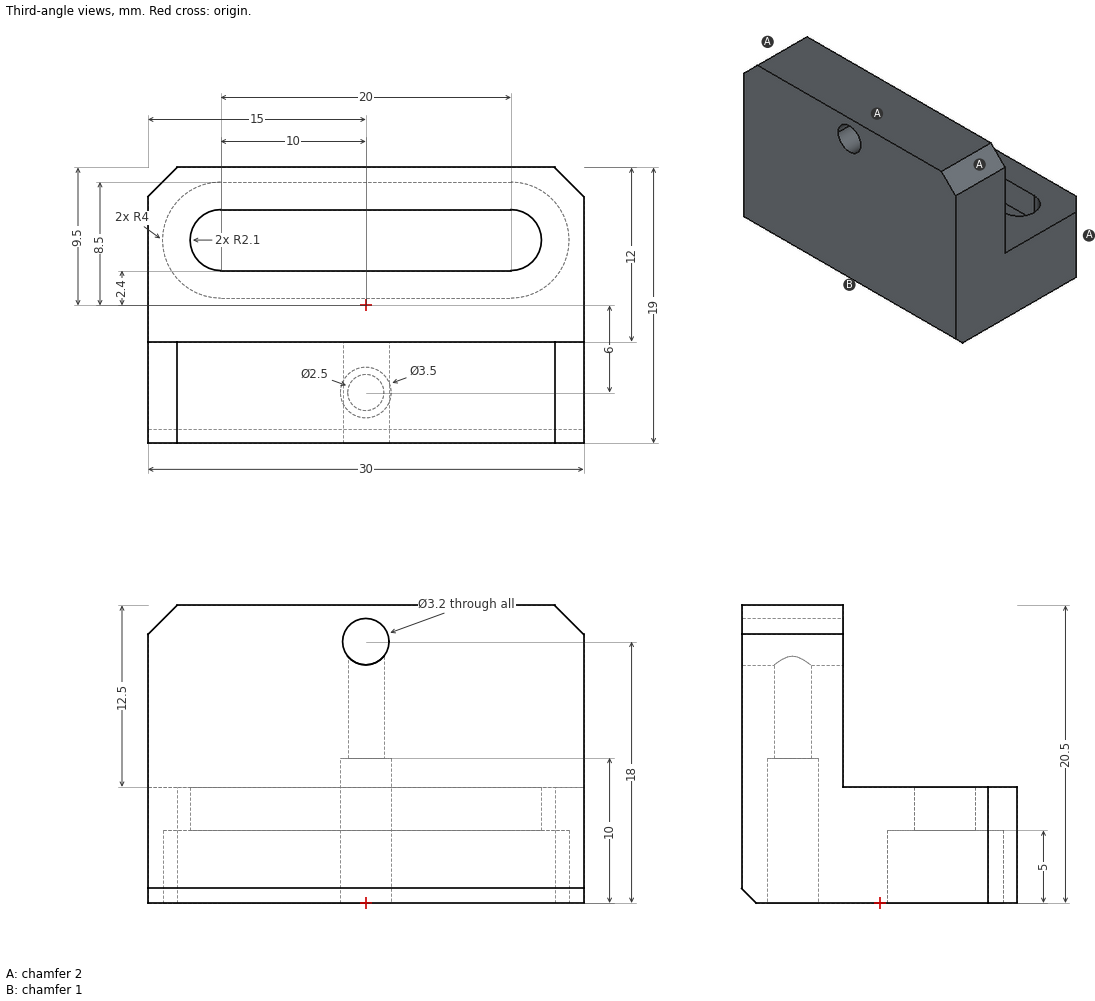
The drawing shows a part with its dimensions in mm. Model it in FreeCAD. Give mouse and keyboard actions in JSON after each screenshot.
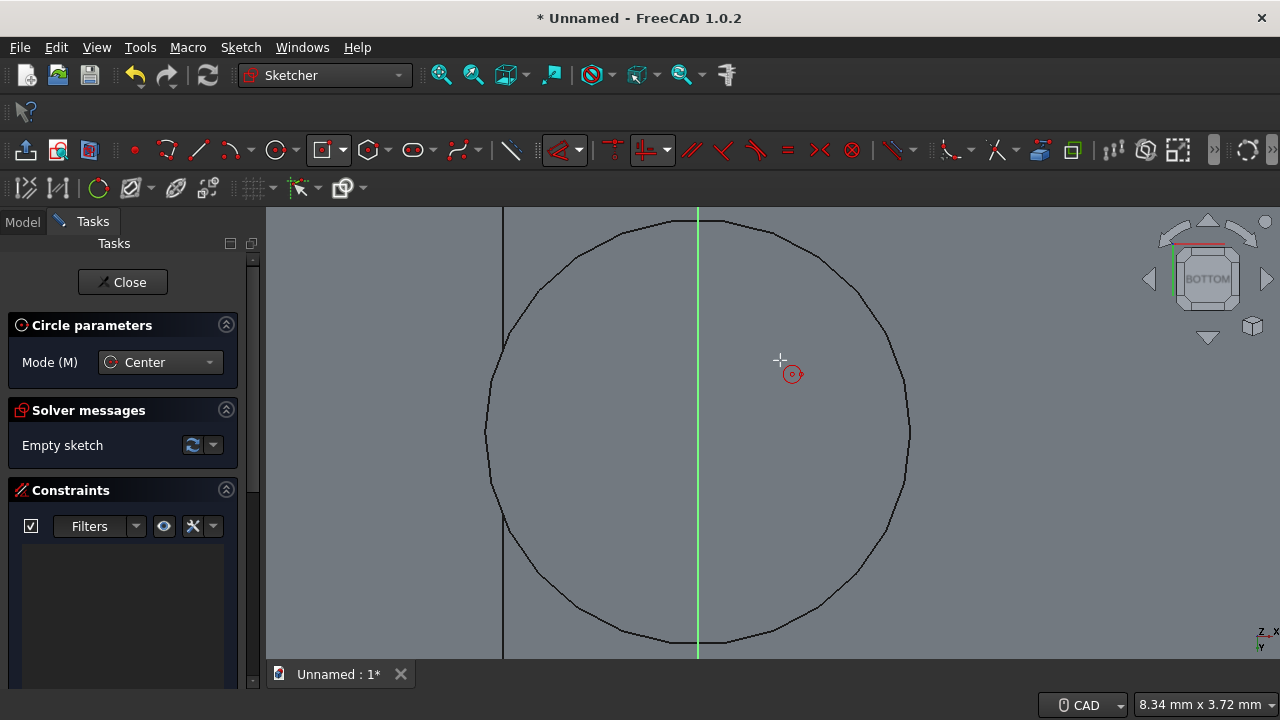
{"action": "left_click", "coordinate": [698, 432]}
{"action": "mouse_move", "coordinate": [805, 325]}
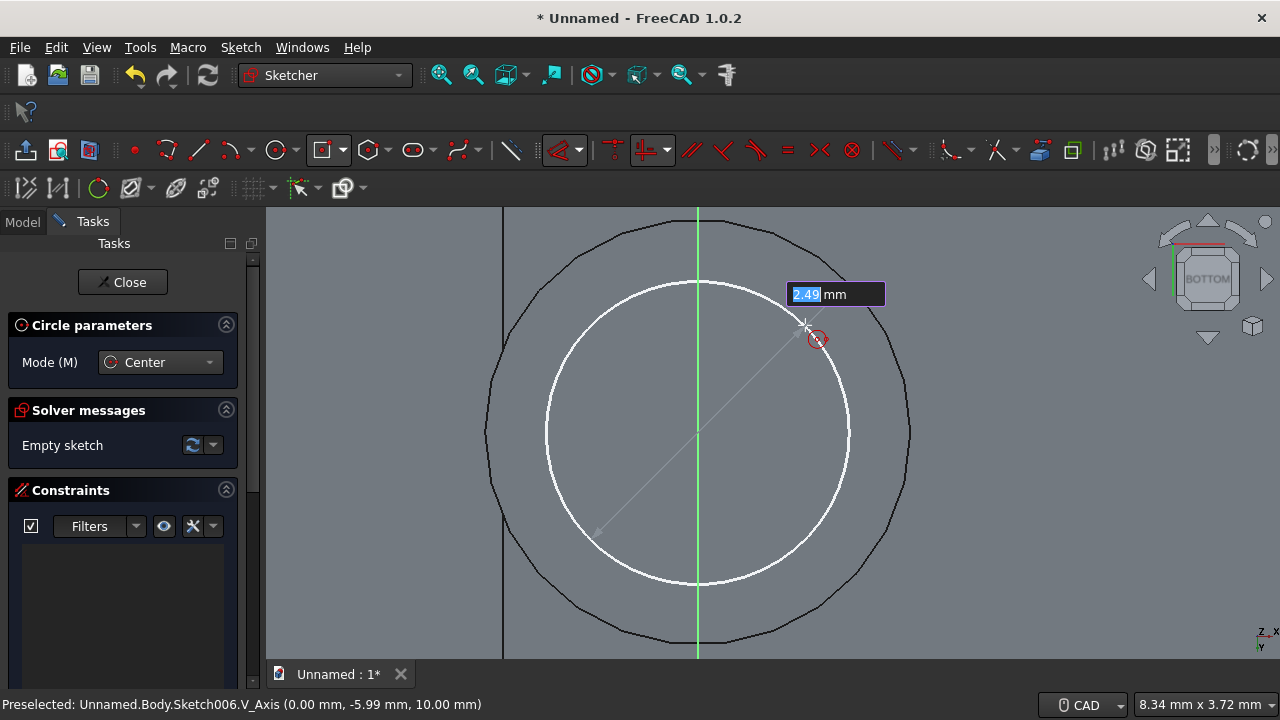
{"action": "type", "text": "2.5"}
{"action": "key", "text": "Return"}
{"action": "key", "text": "Escape"}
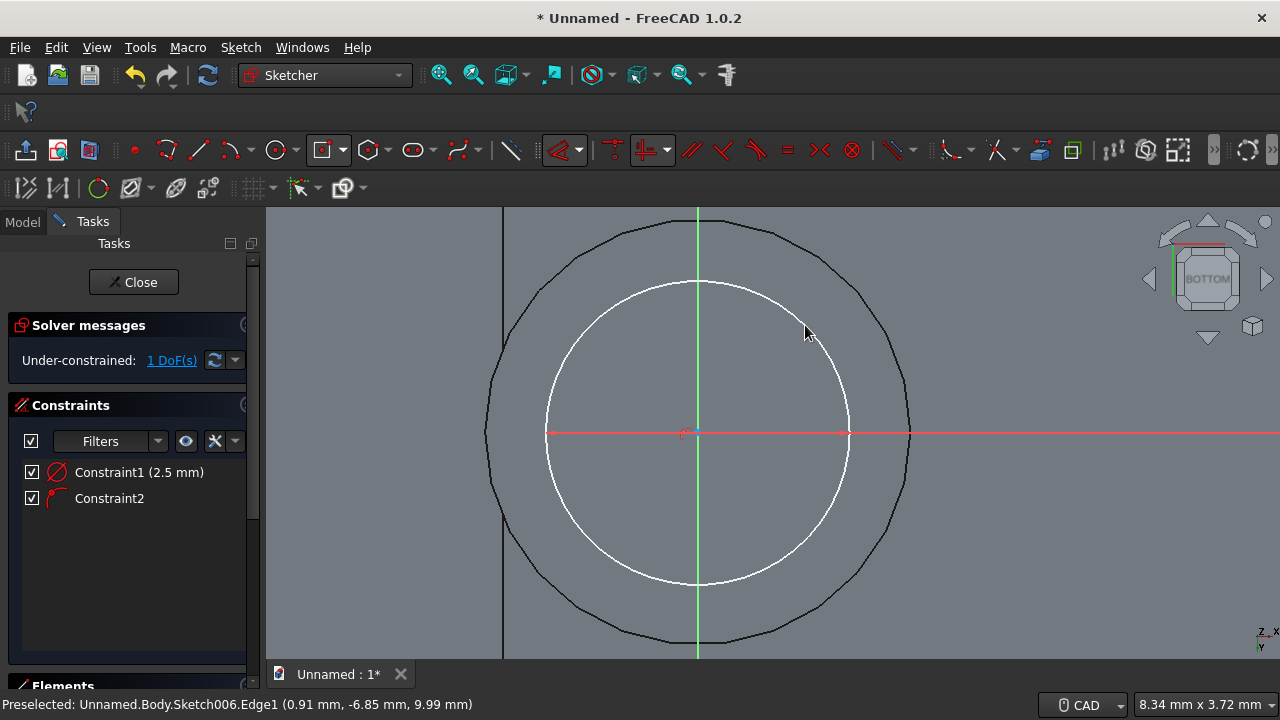
{"action": "left_click", "coordinate": [698, 433]}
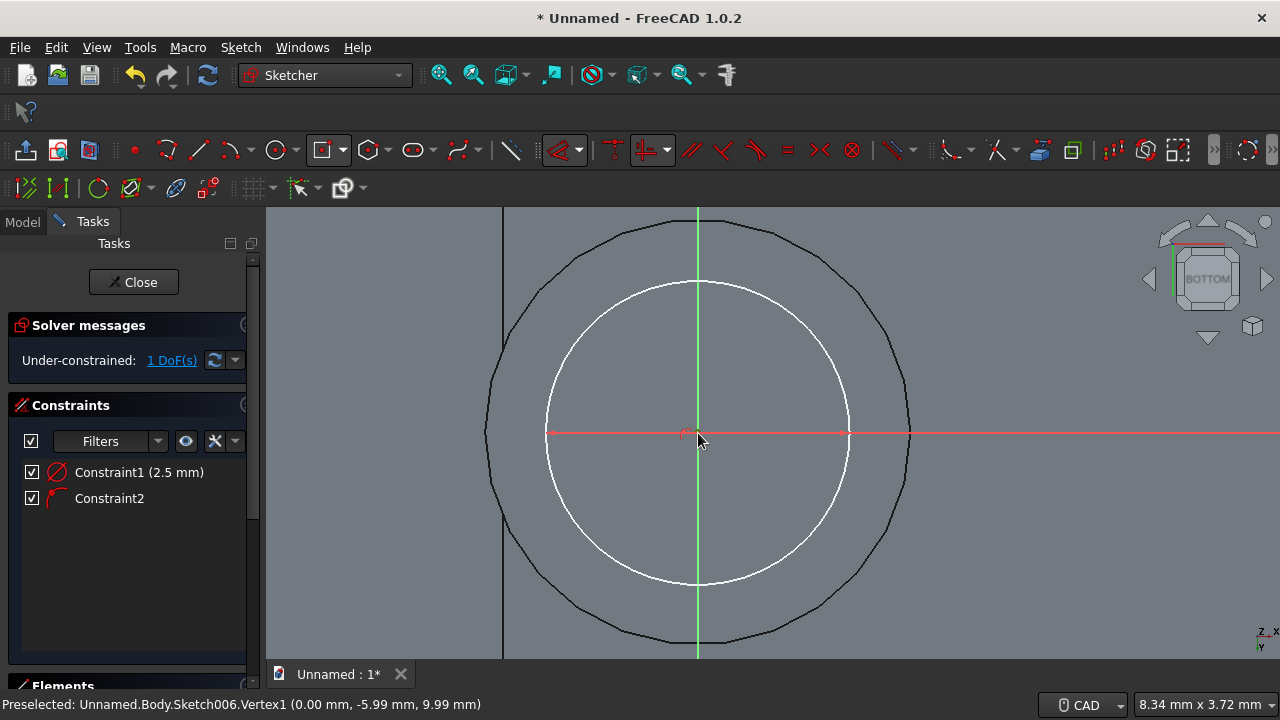
{"action": "key", "text": "i"}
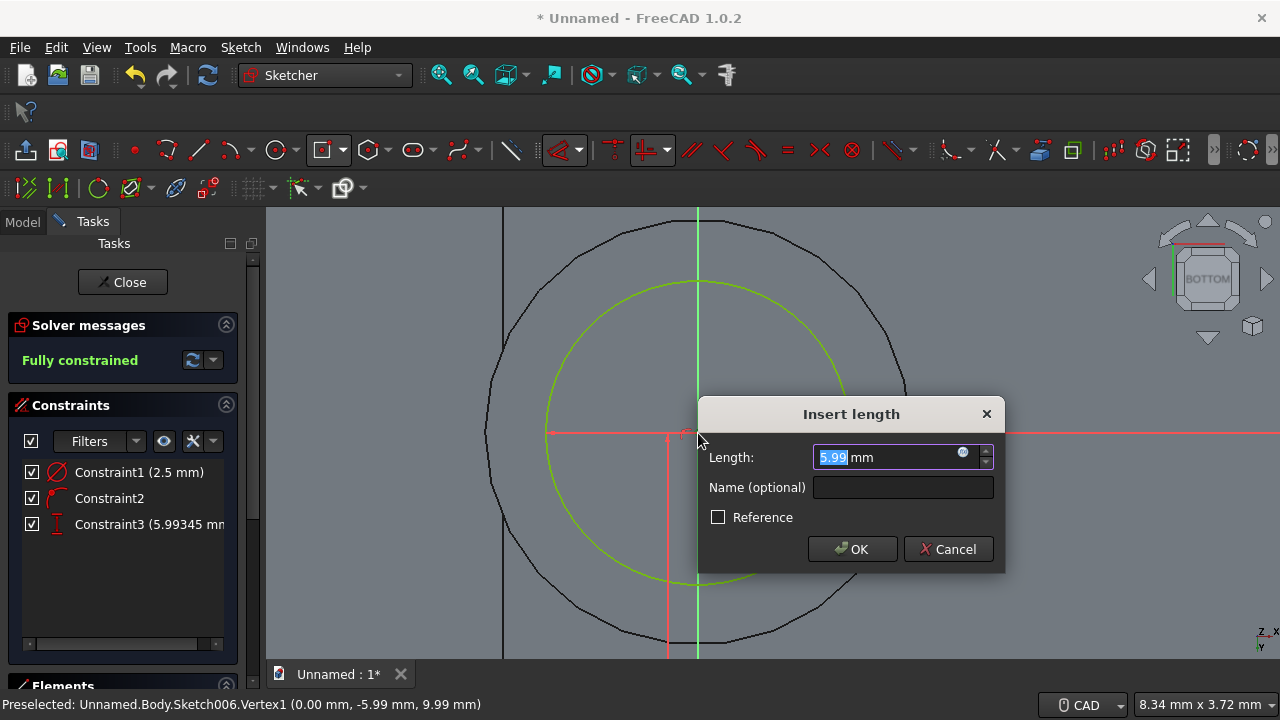
{"action": "type", "text": "6"}
{"action": "key", "text": "Return"}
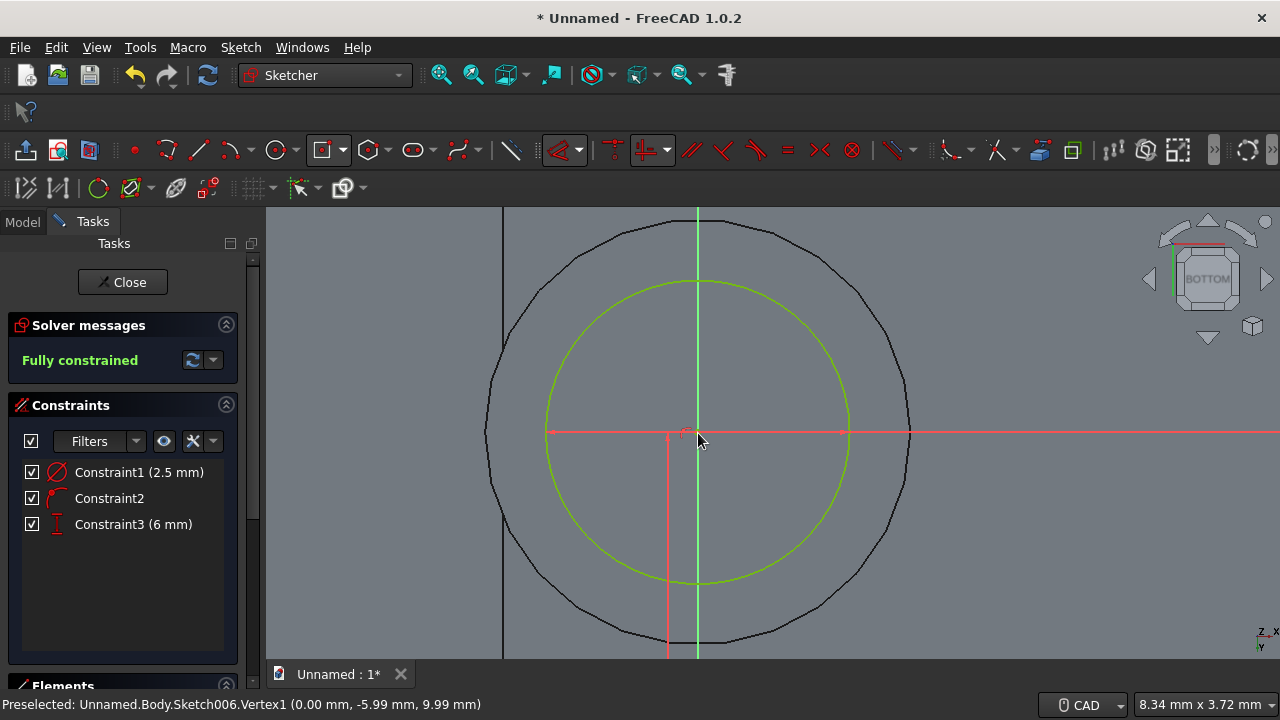
{"action": "left_click", "coordinate": [123, 282]}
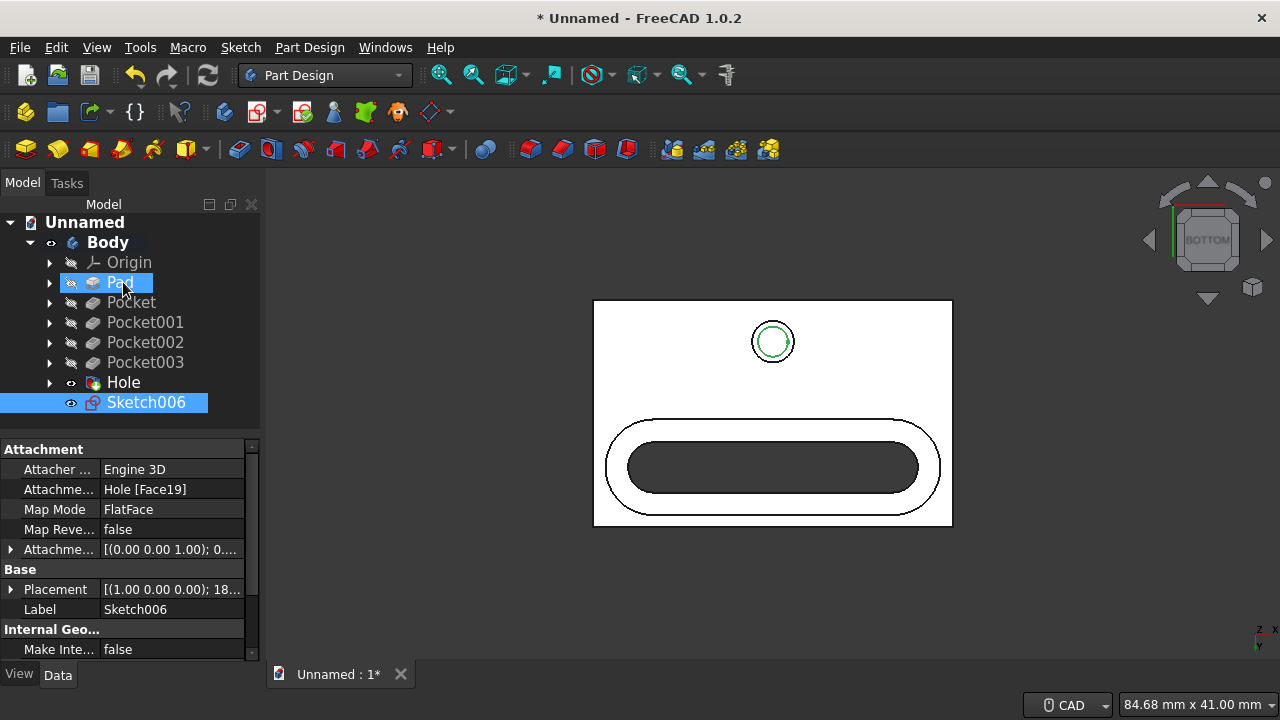
{"action": "left_click", "coordinate": [240, 150]}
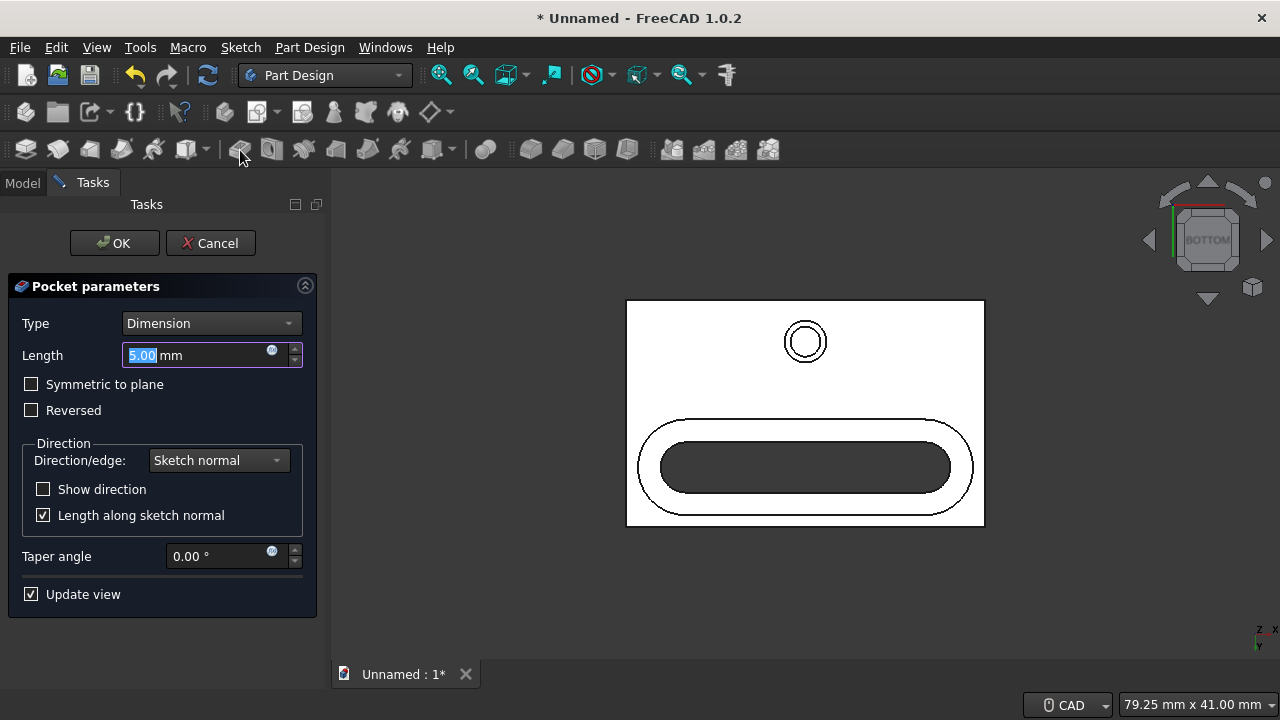
{"action": "left_click", "coordinate": [212, 324]}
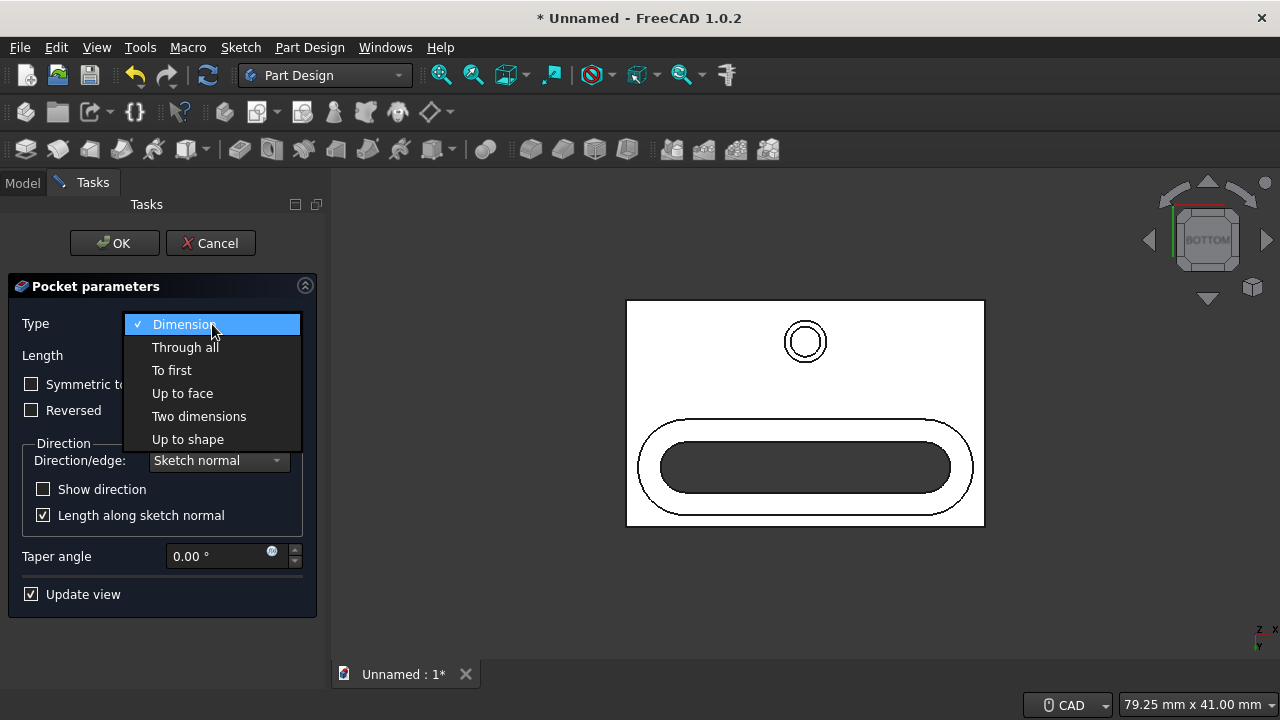
{"action": "left_click", "coordinate": [212, 370]}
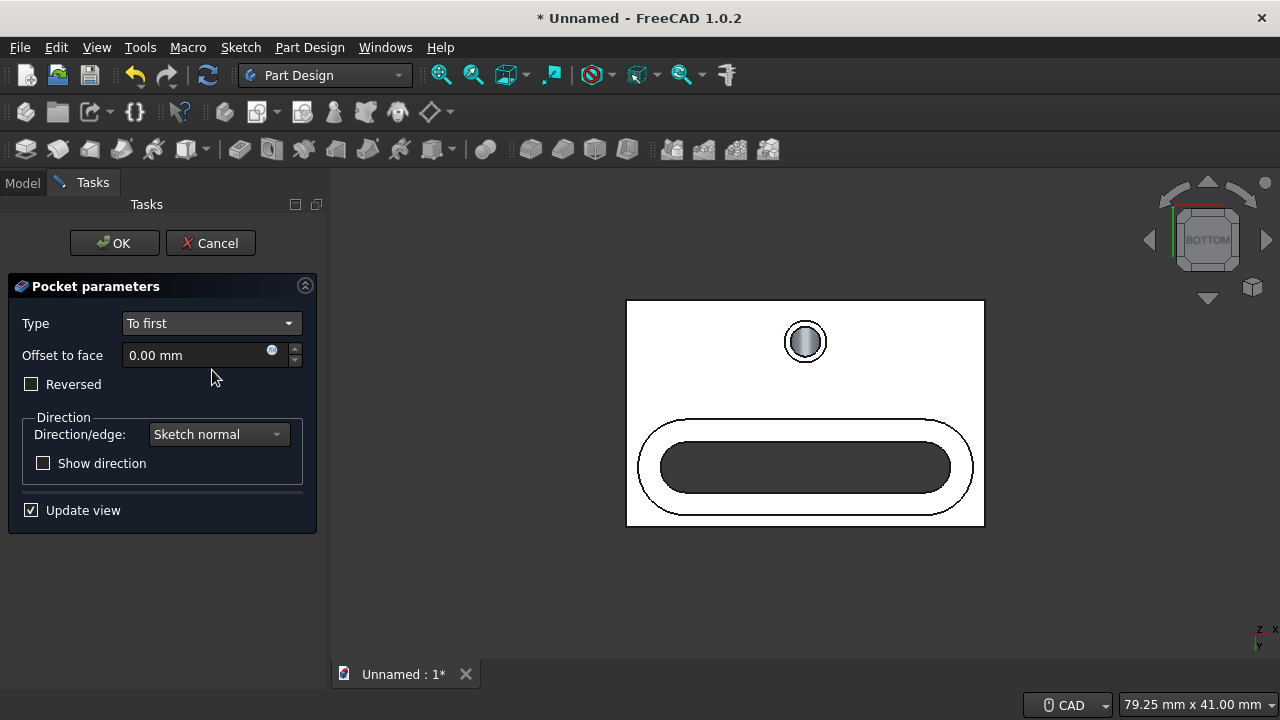
{"action": "left_click", "coordinate": [115, 243]}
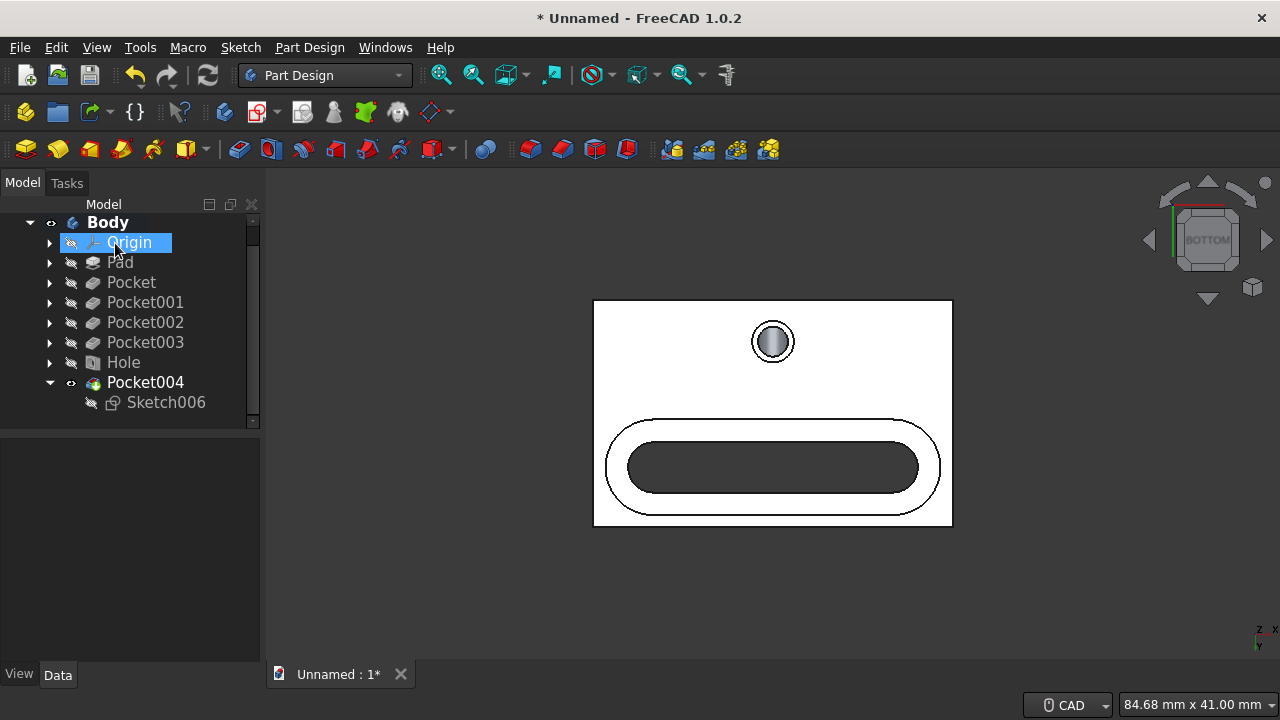
{"action": "key", "text": "0"}